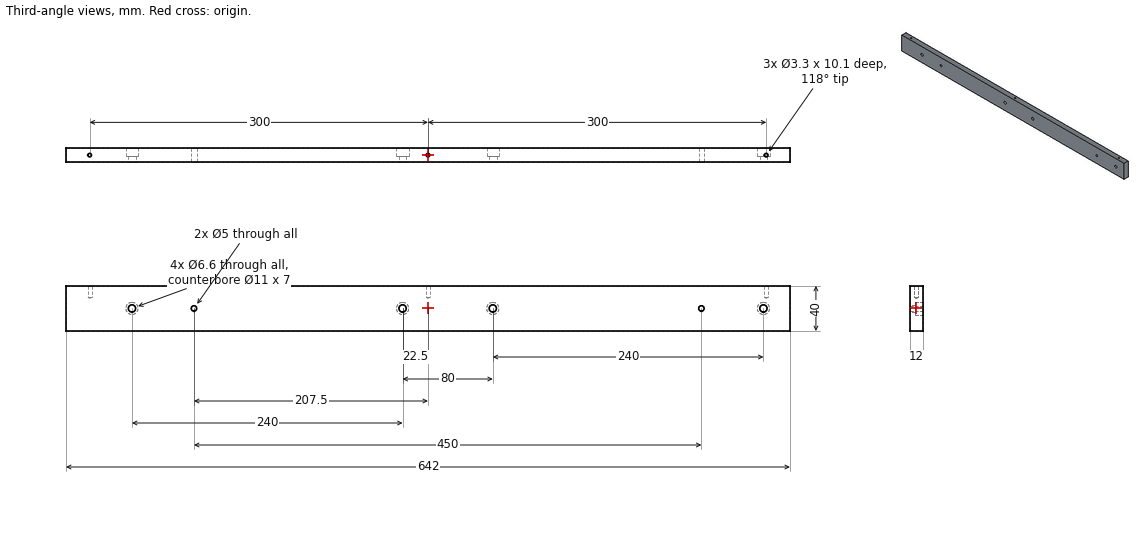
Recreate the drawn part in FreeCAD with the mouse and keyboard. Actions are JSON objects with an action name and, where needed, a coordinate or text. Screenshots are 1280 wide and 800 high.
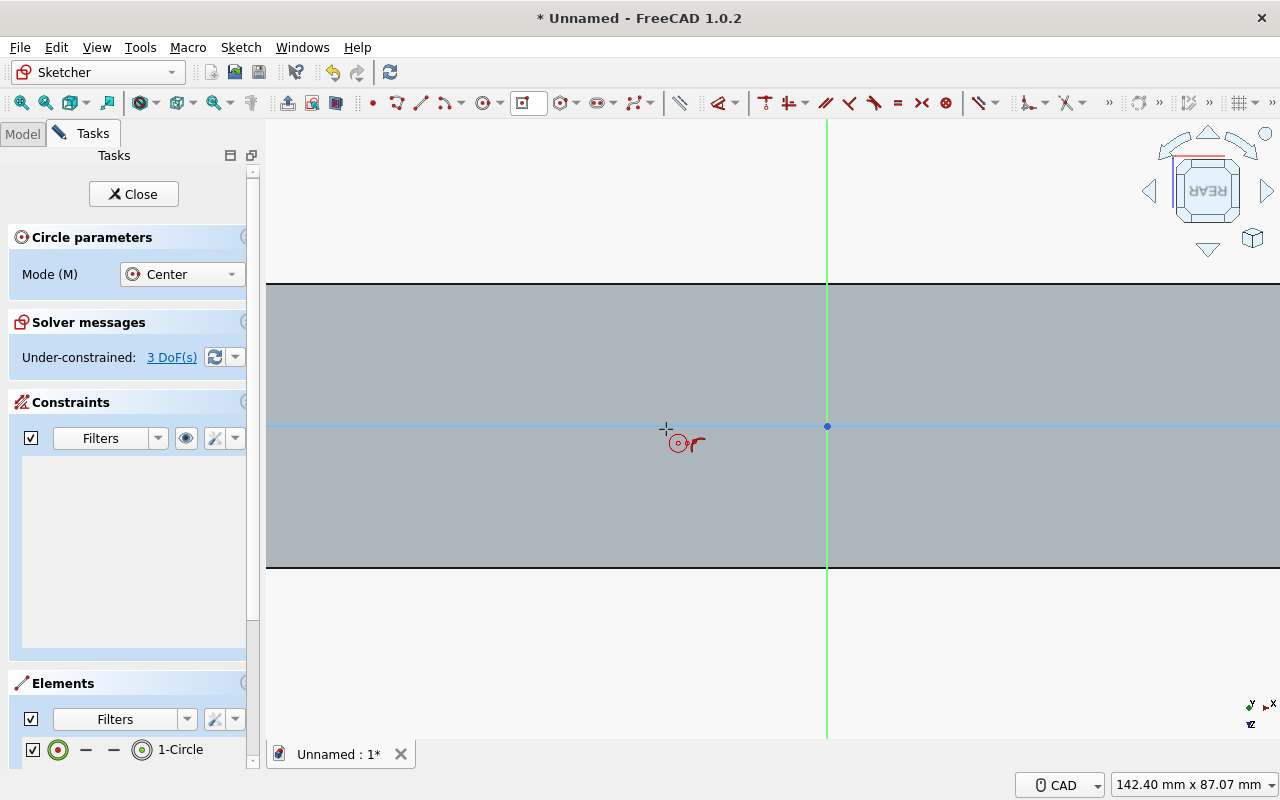
{"action": "scroll", "coordinate": [666, 429], "scroll_direction": "down", "scroll_amount": 10}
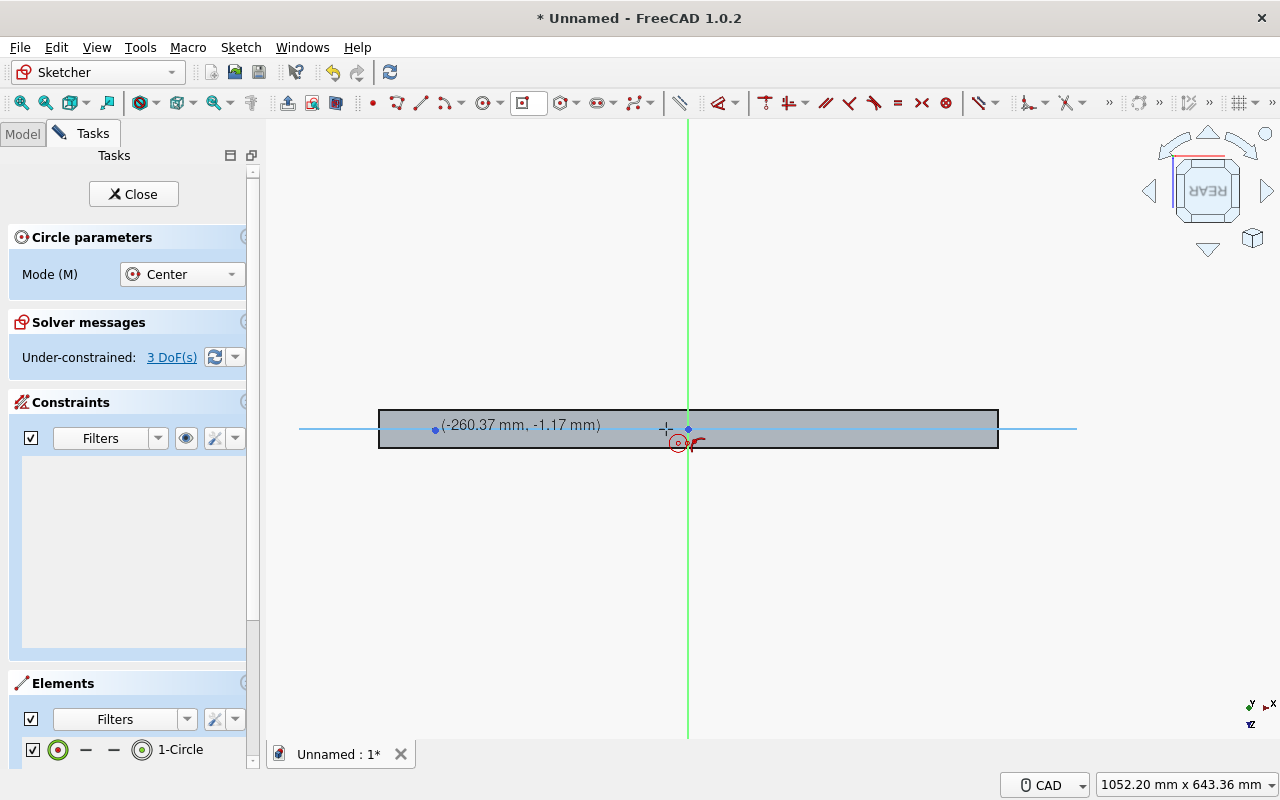
{"action": "left_click", "coordinate": [666, 429]}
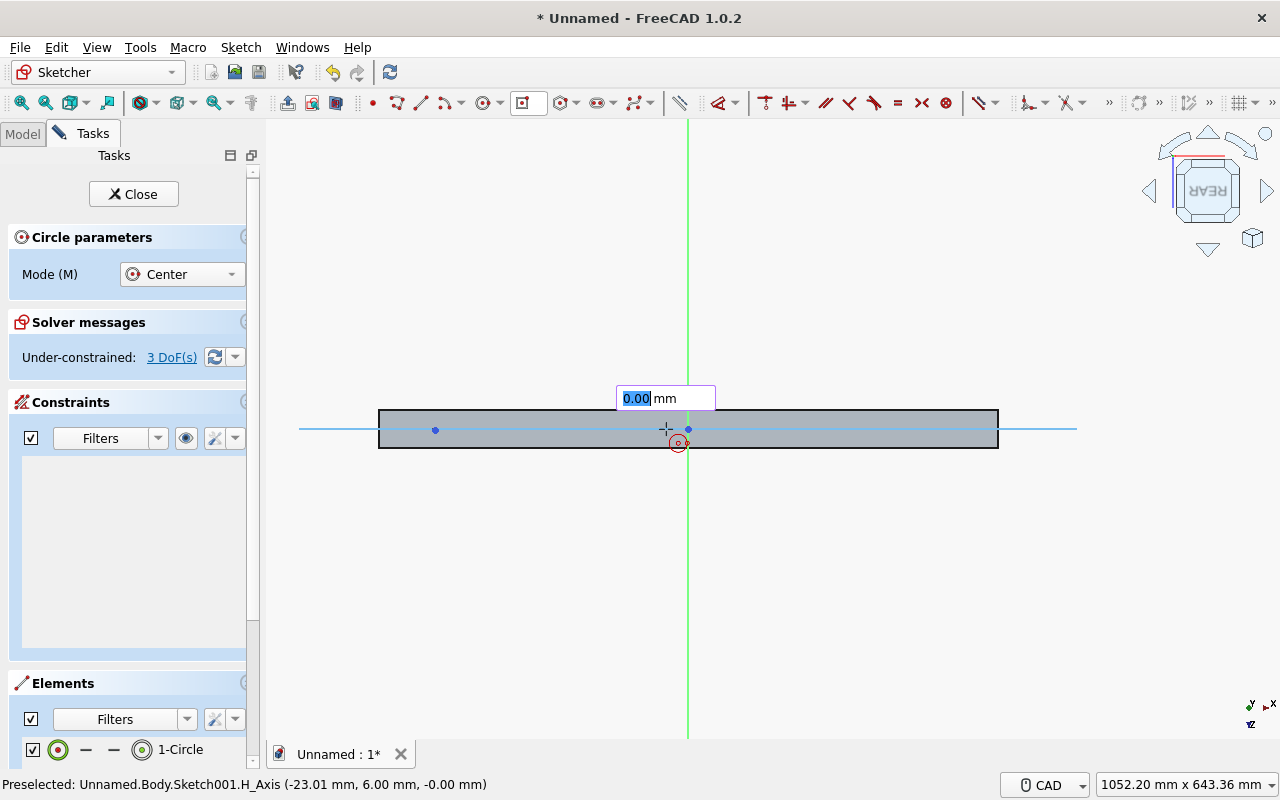
{"action": "scroll", "coordinate": [665, 432], "scroll_direction": "up", "scroll_amount": 9}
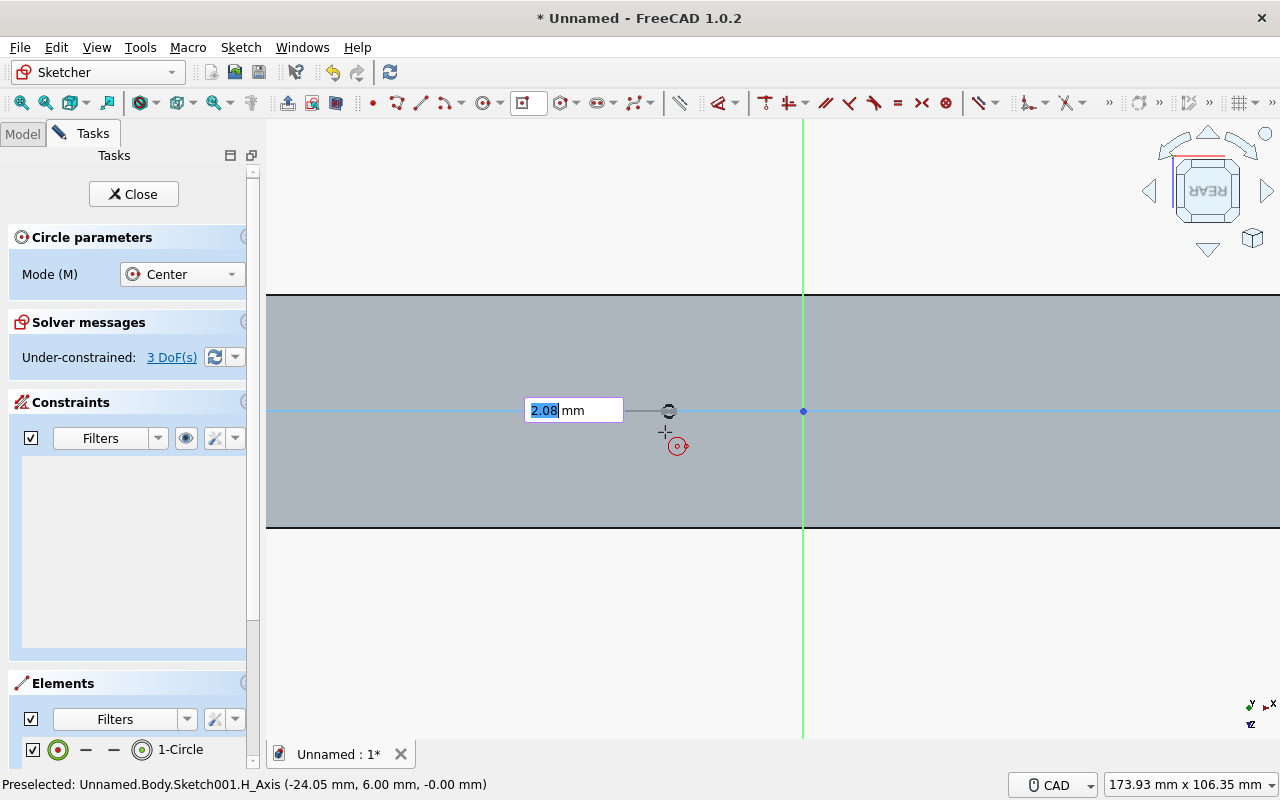
{"action": "left_click", "coordinate": [665, 430]}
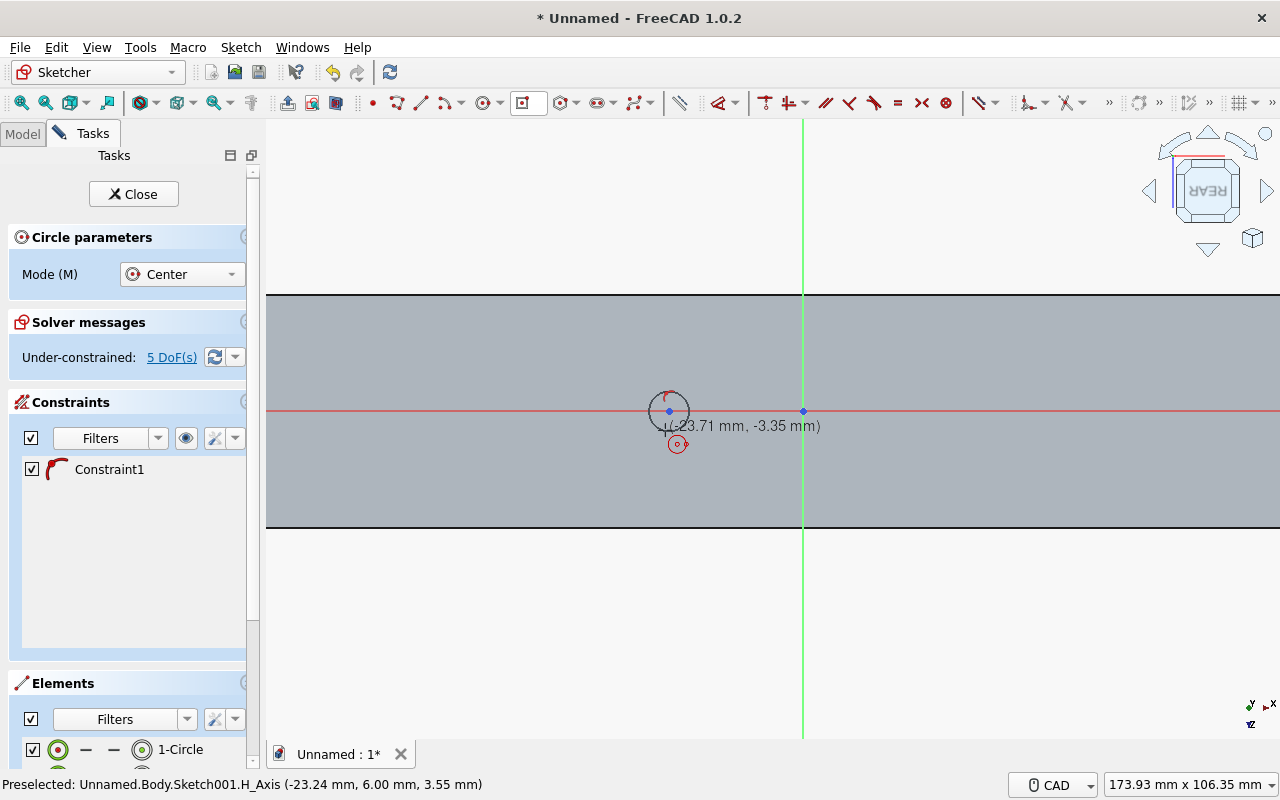
{"action": "scroll", "coordinate": [665, 432], "scroll_direction": "down", "scroll_amount": 9}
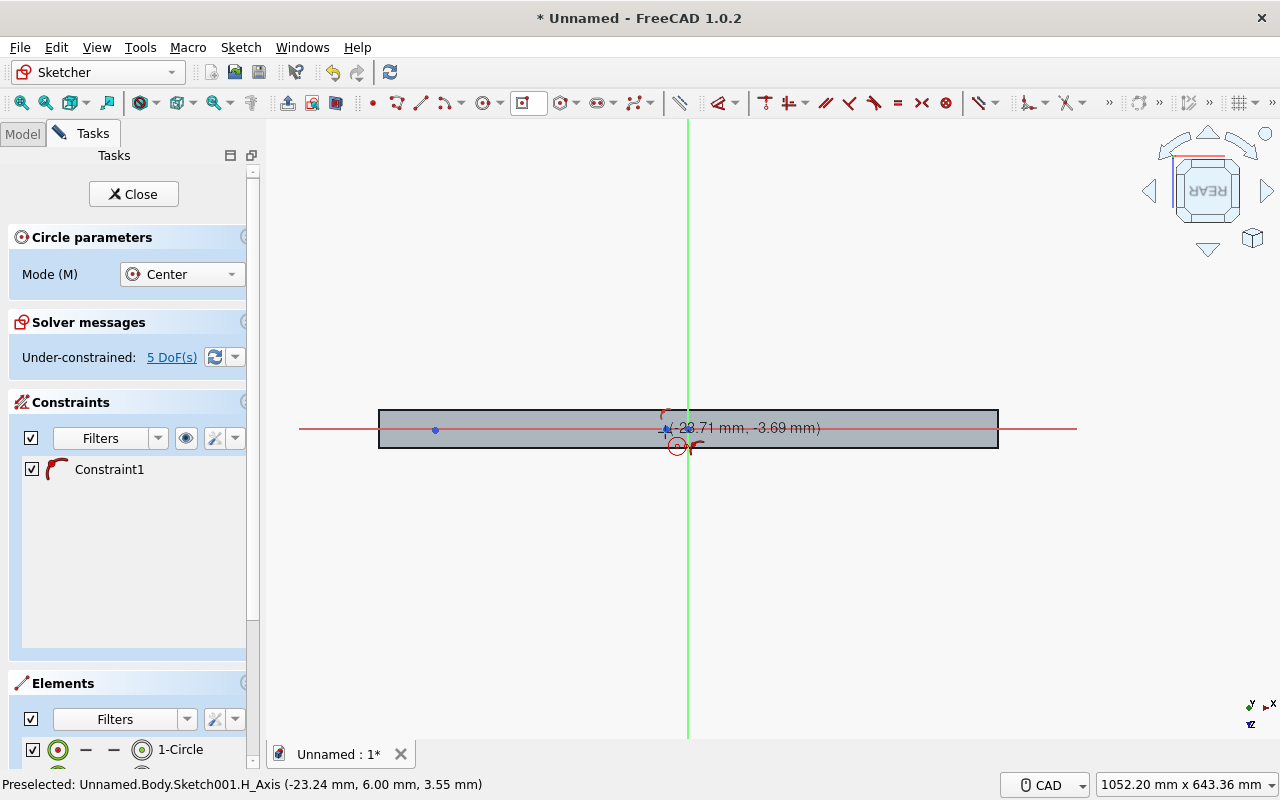
{"action": "scroll", "coordinate": [744, 429], "scroll_direction": "up", "scroll_amount": 10}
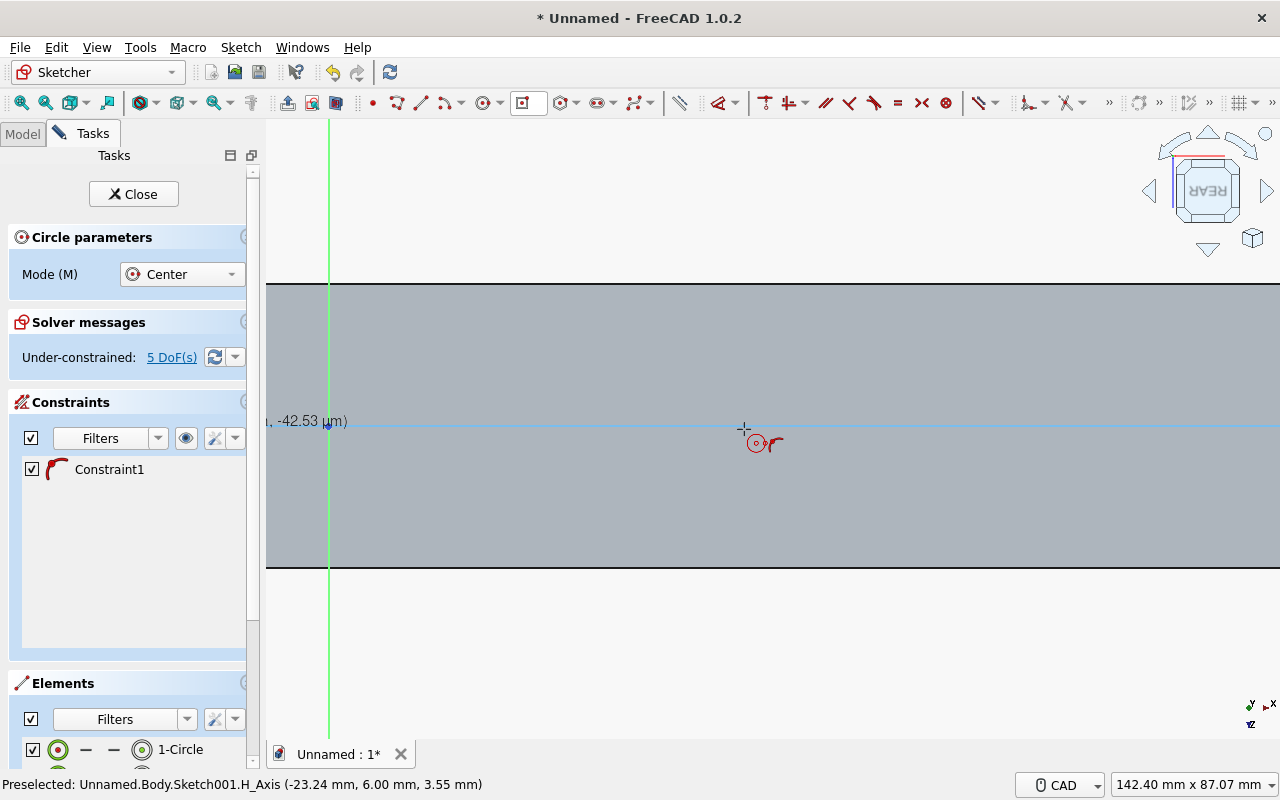
{"action": "scroll", "coordinate": [744, 429], "scroll_direction": "down", "scroll_amount": 10}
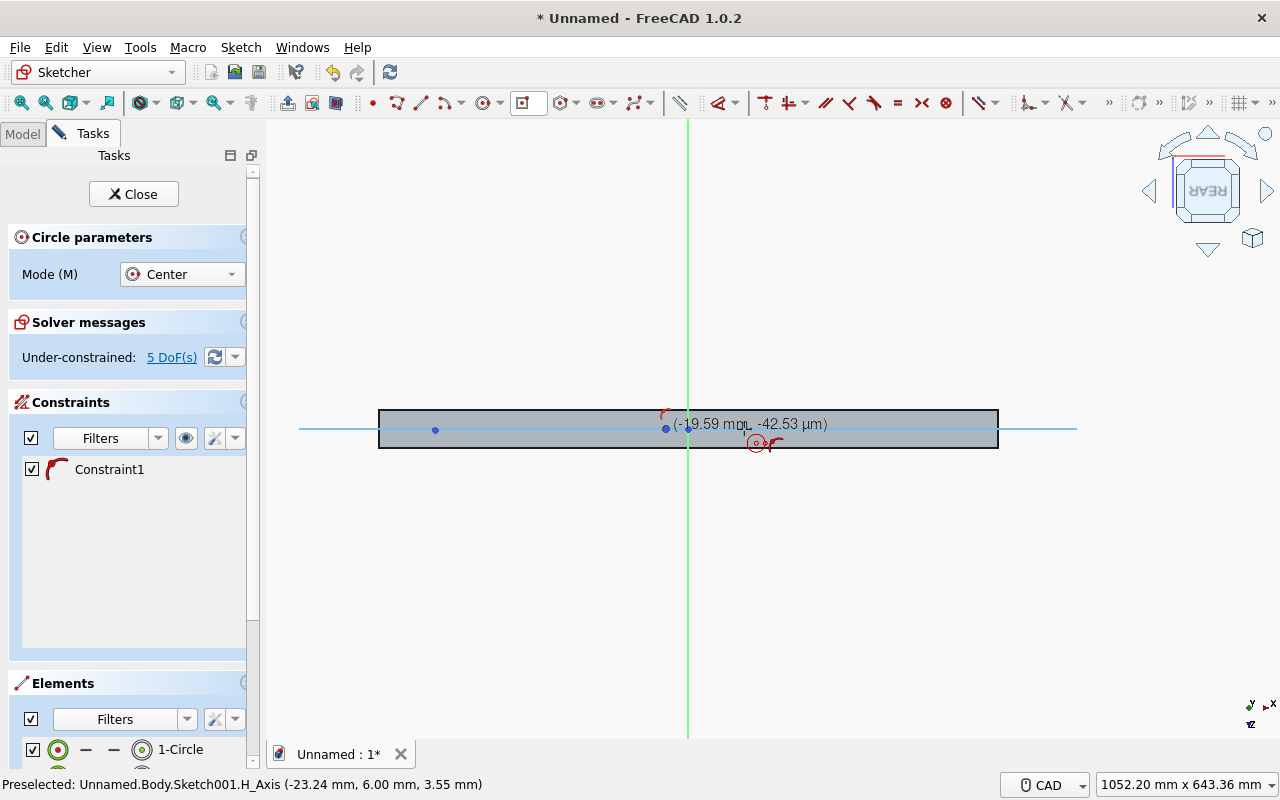
{"action": "left_click", "coordinate": [744, 429]}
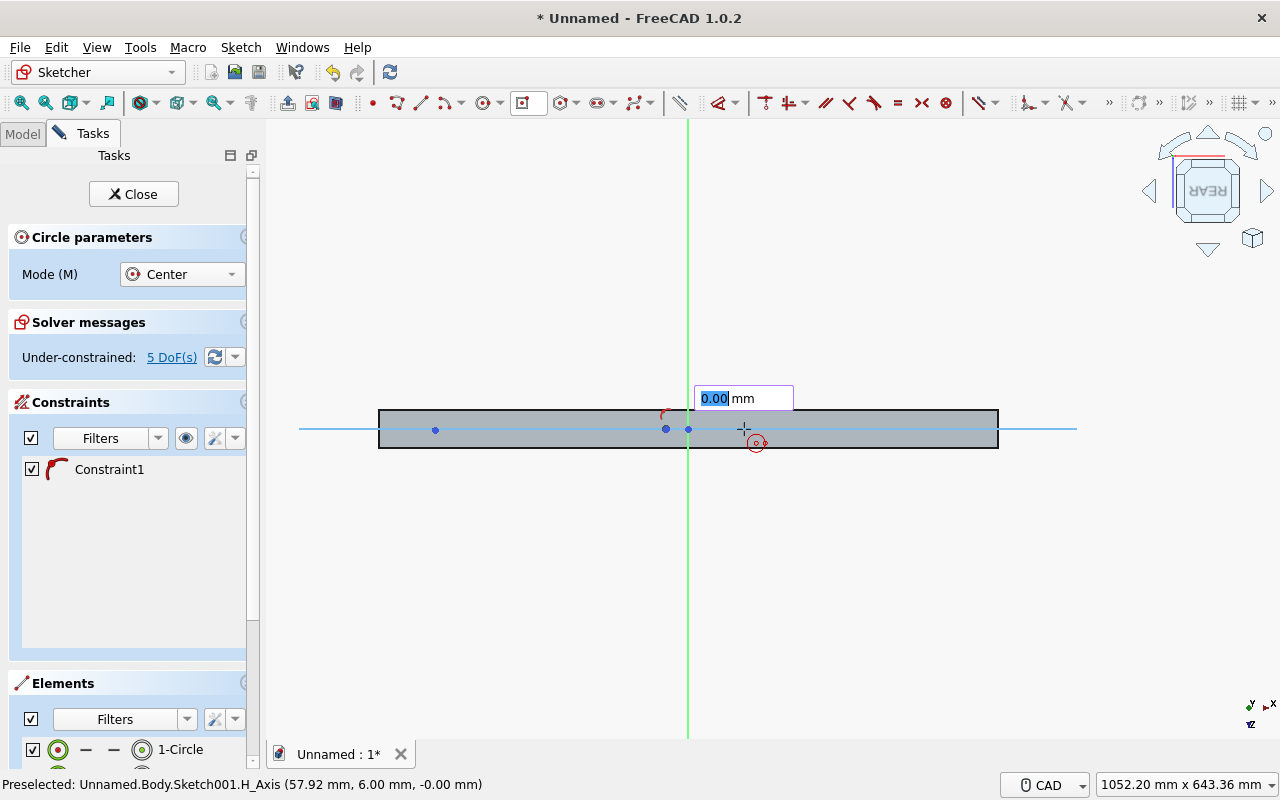
{"action": "scroll", "coordinate": [743, 432], "scroll_direction": "up", "scroll_amount": 9}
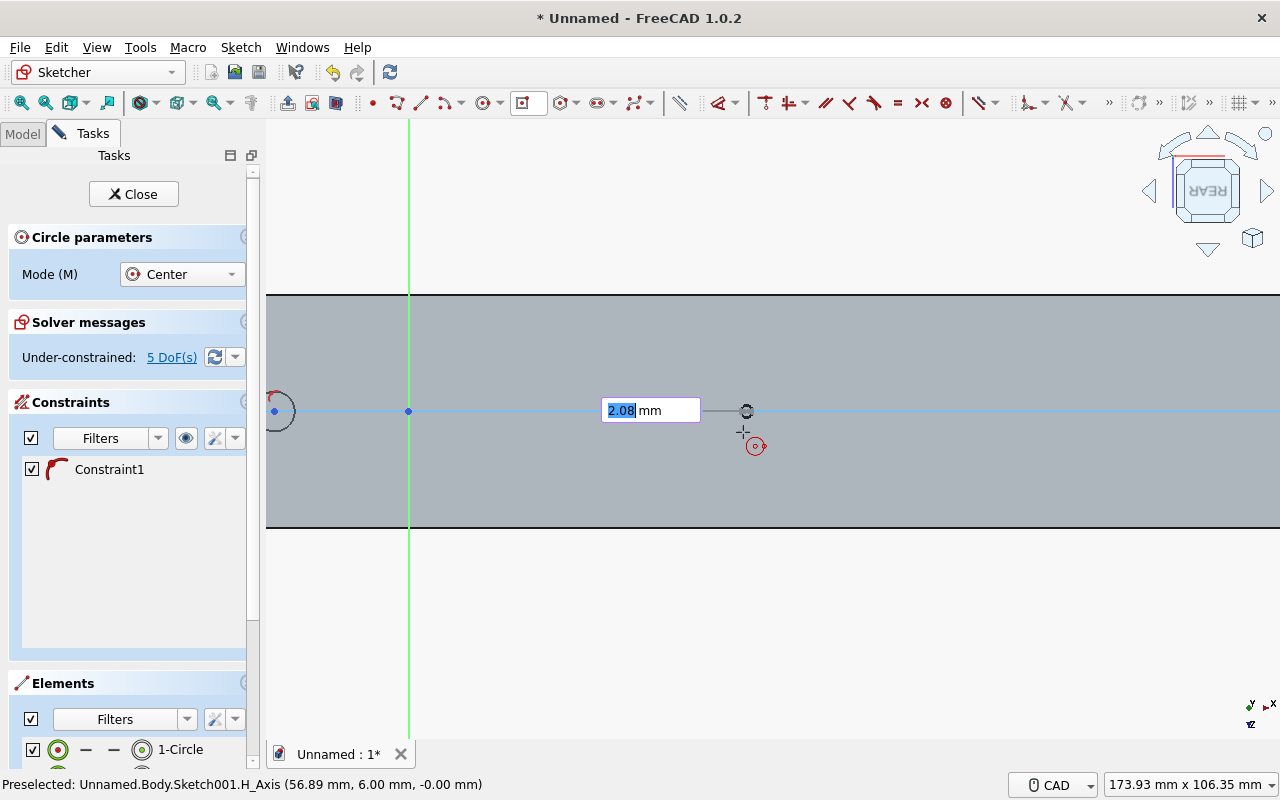
{"action": "left_click", "coordinate": [738, 430]}